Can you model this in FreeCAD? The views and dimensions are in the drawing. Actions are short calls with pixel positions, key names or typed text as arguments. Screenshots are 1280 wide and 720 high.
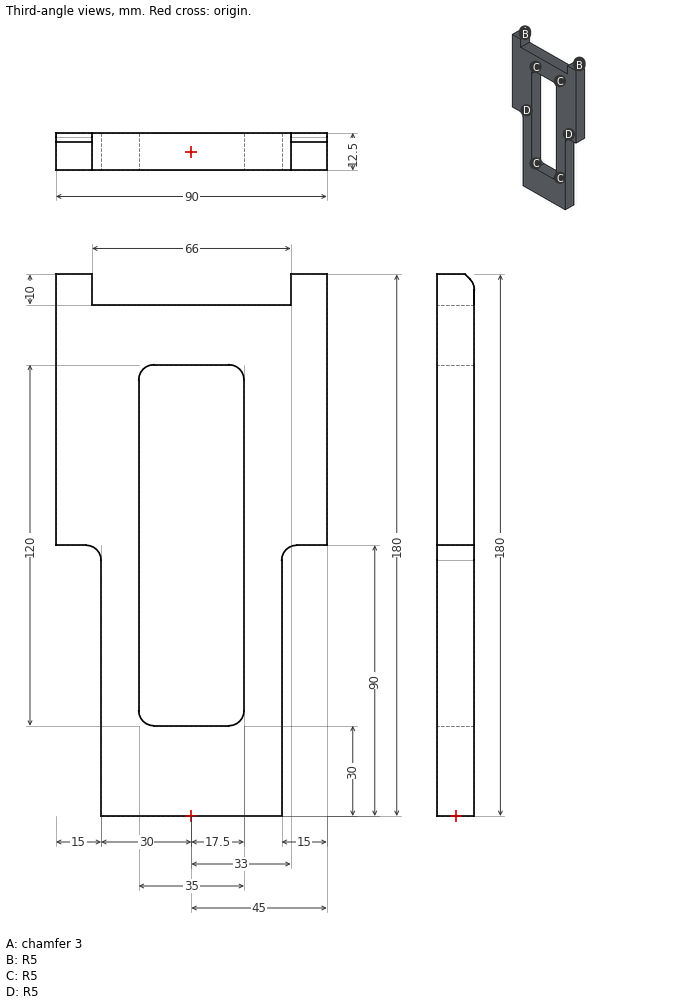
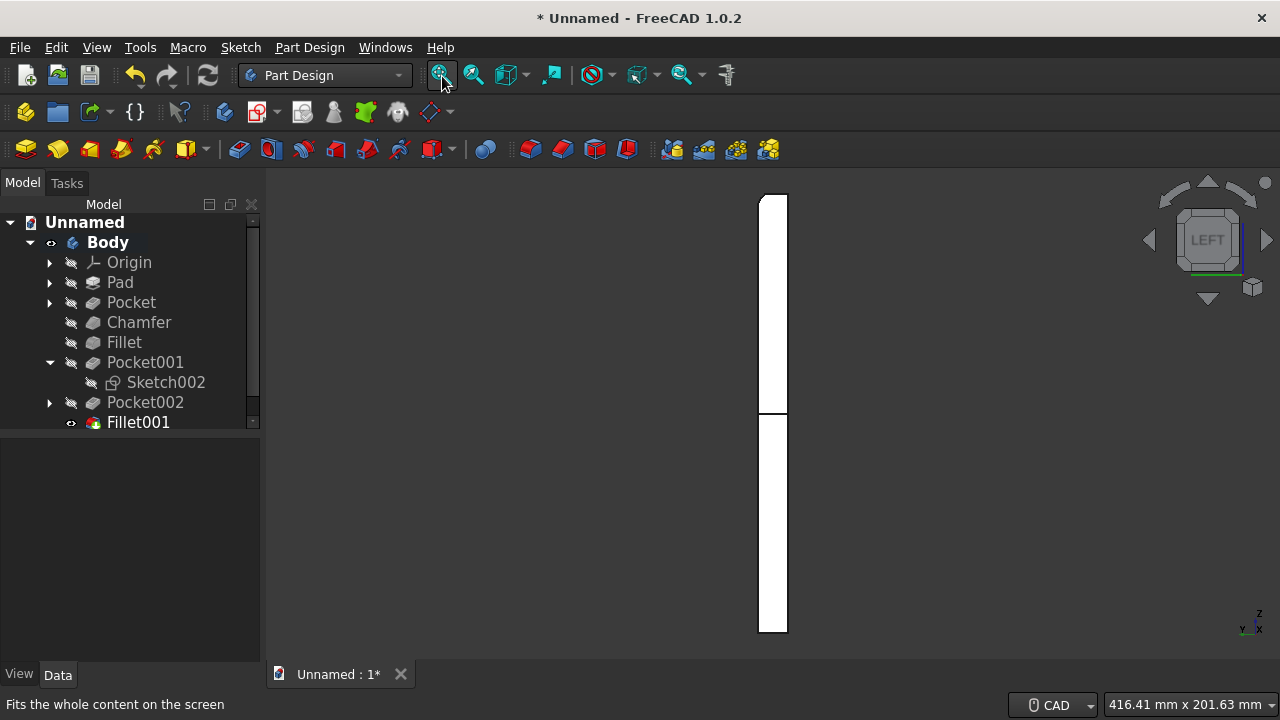
key(v)
key(3)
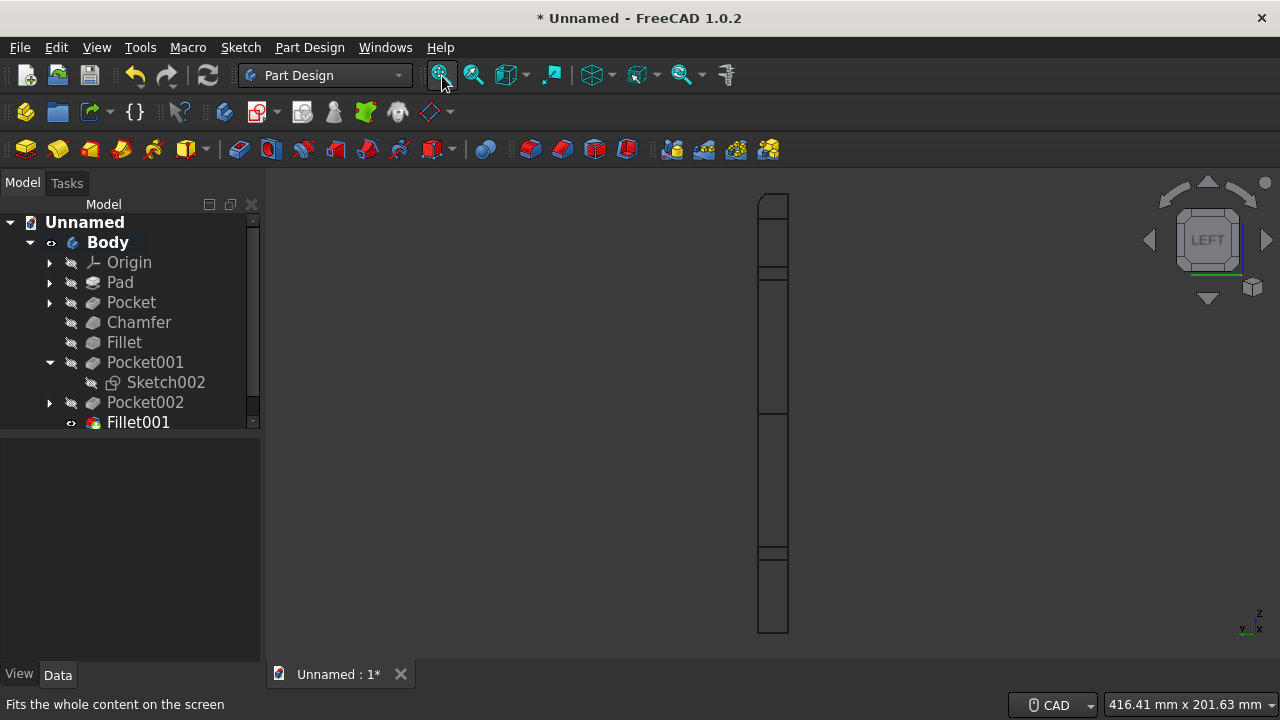
key(0)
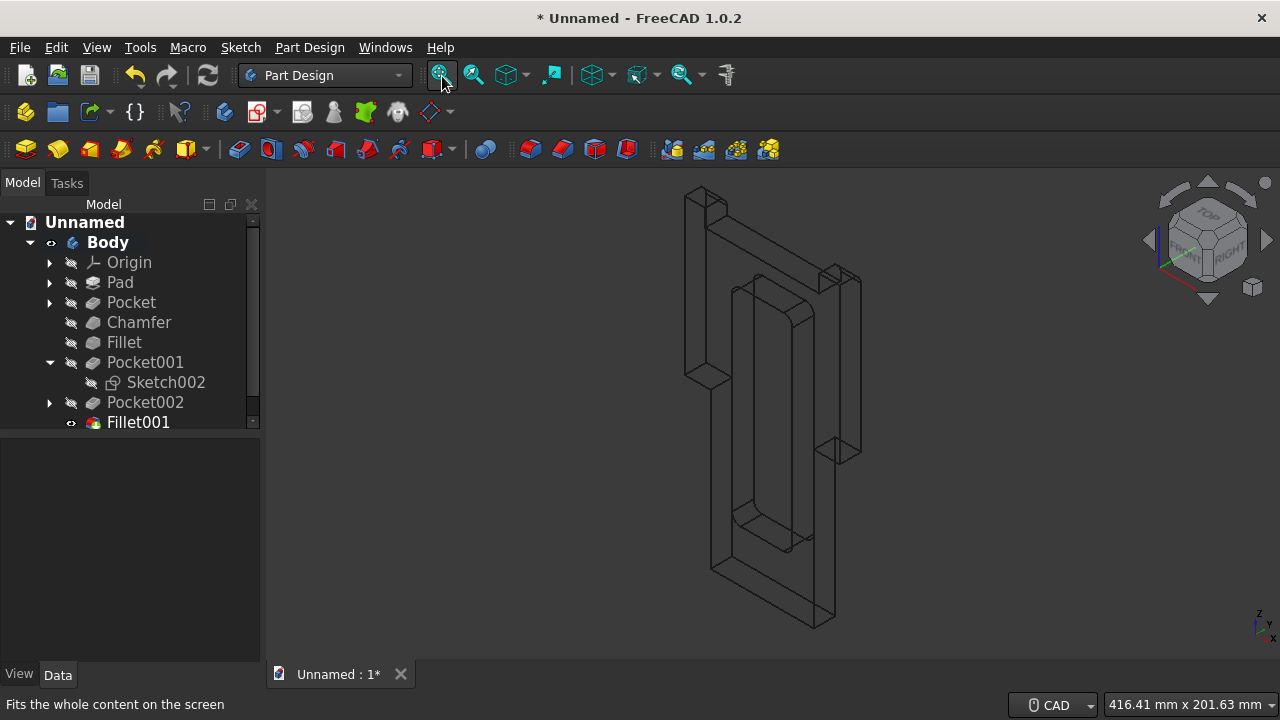
click(825, 442)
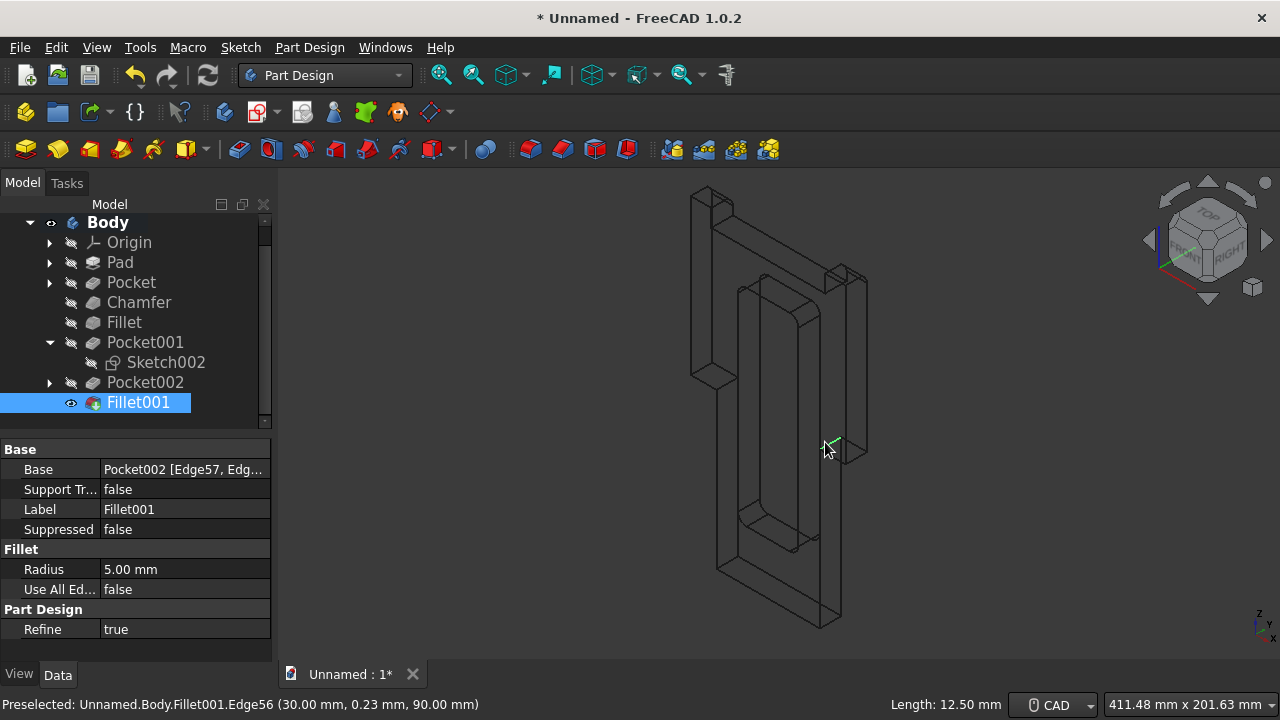
click(727, 383, ctrl)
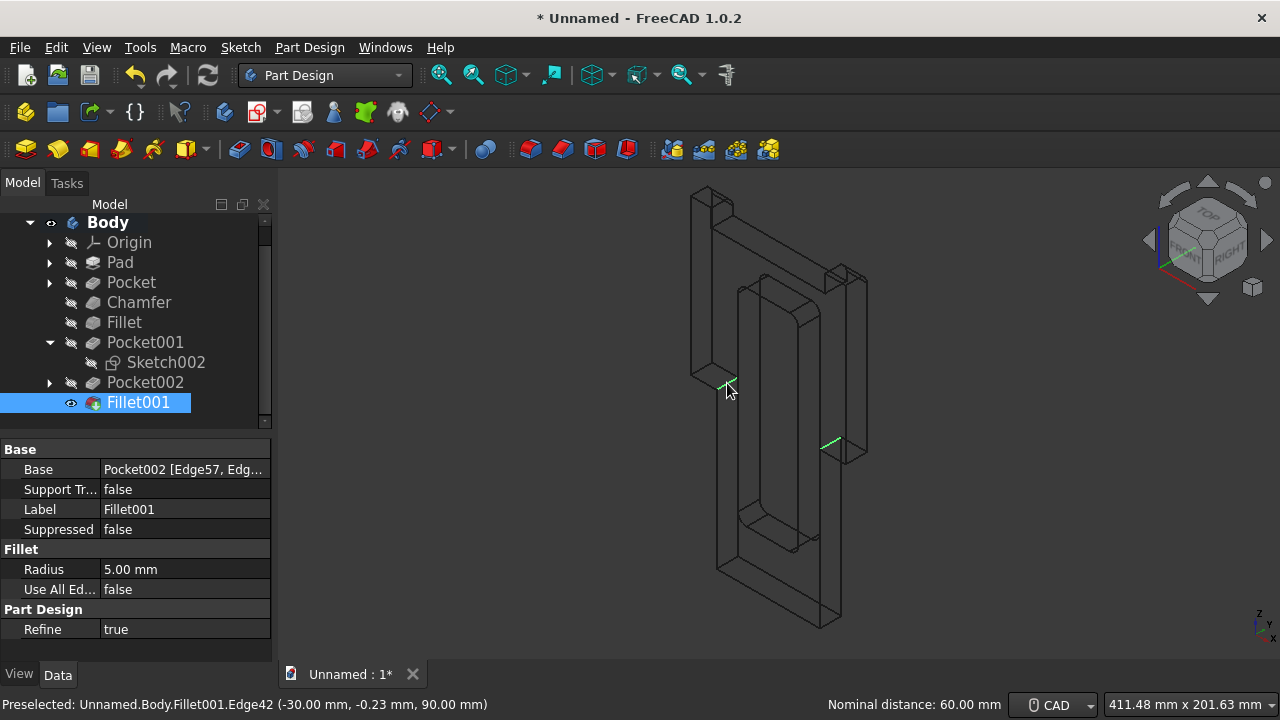
key(v)
key(1)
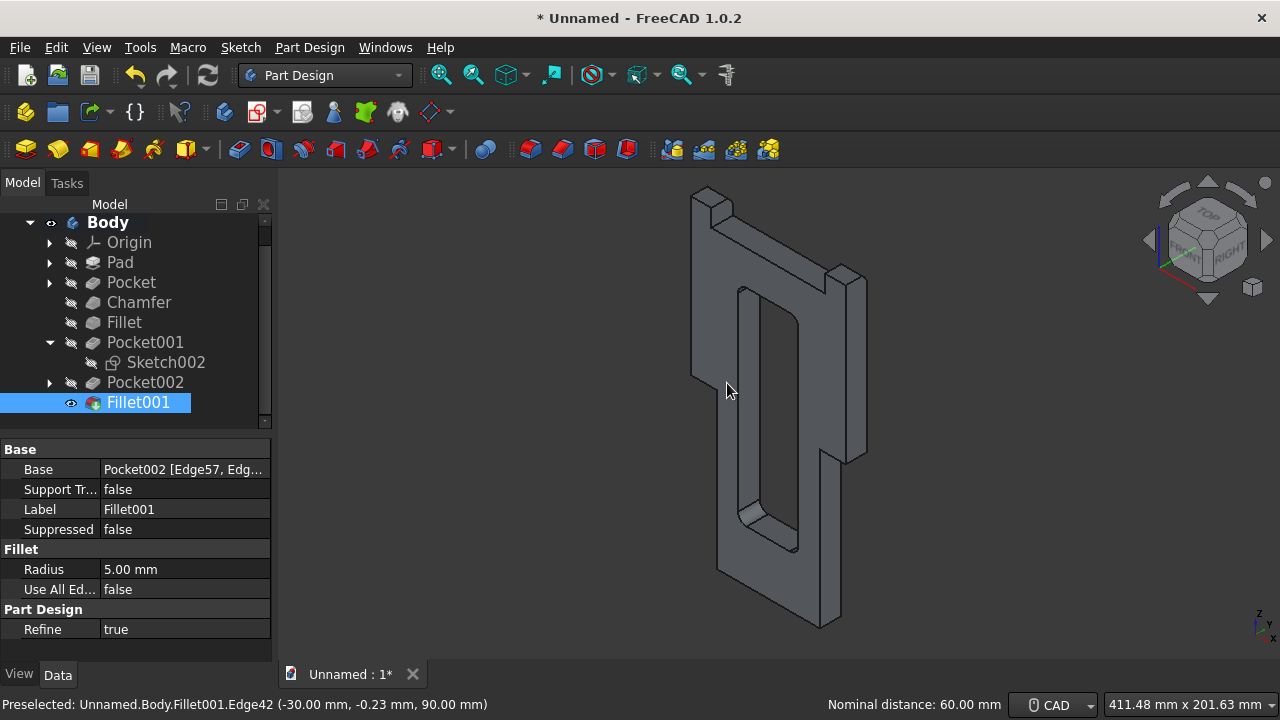
click(532, 150)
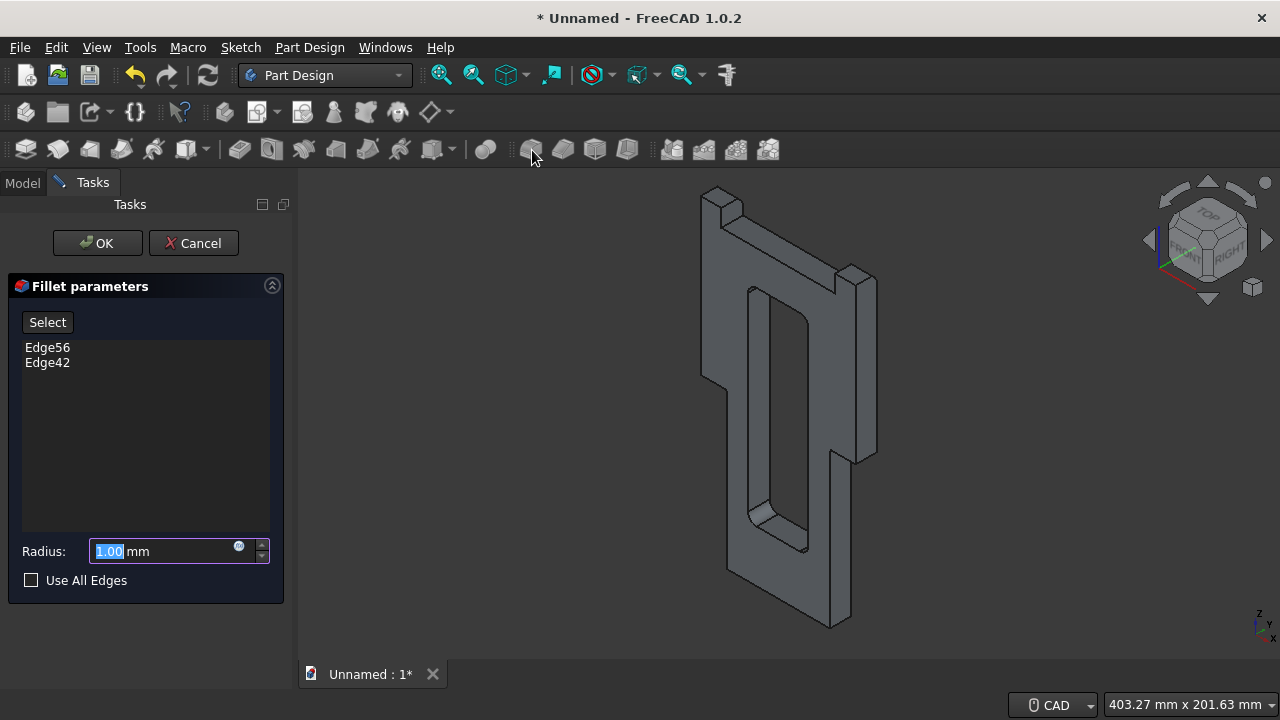
text(5)
key(Tab)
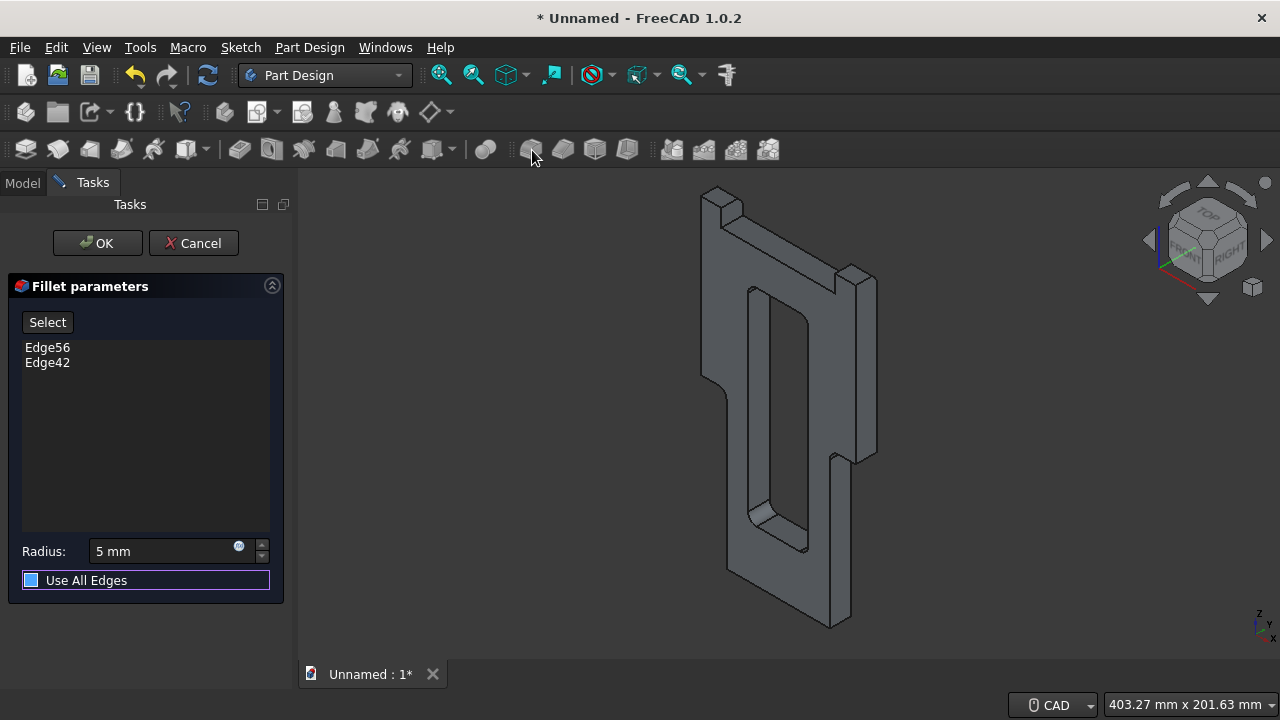
click(98, 243)